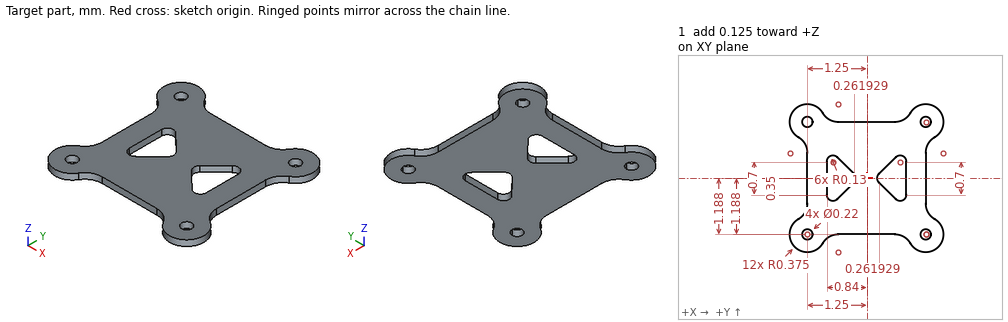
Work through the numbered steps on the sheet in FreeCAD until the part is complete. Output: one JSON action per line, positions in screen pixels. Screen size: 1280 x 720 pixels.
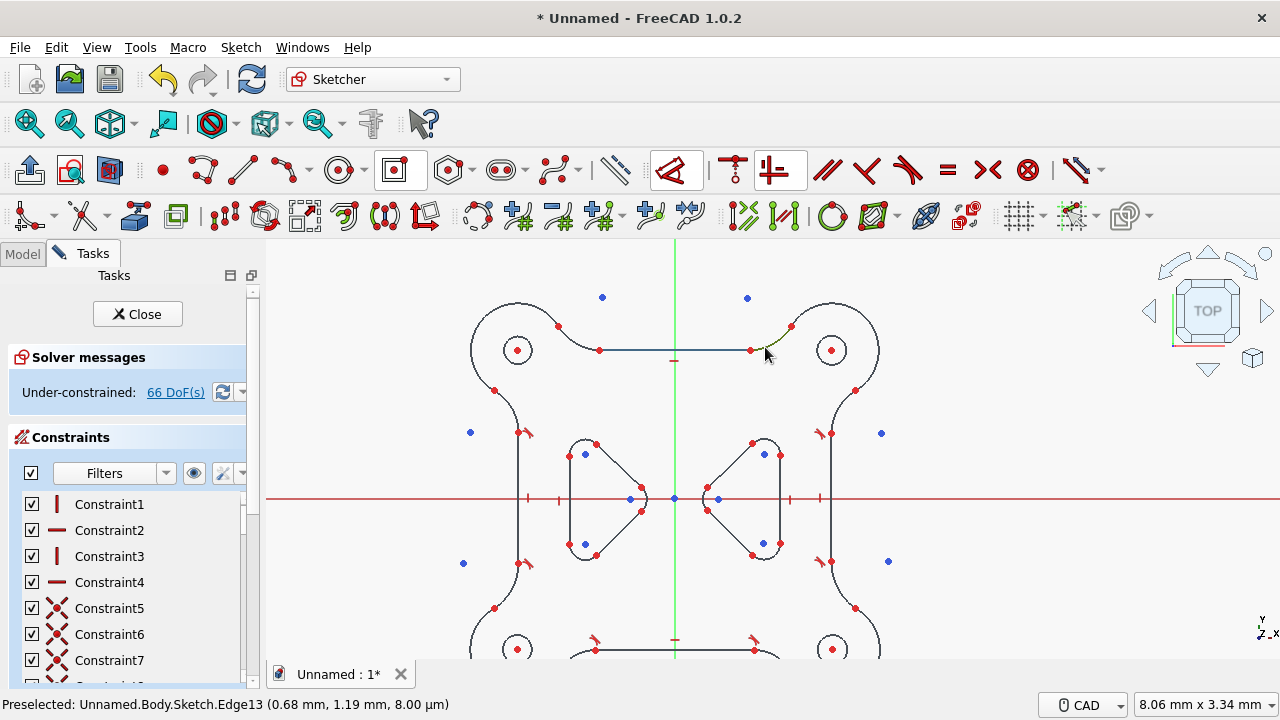
{"action": "left_click", "coordinate": [908, 170]}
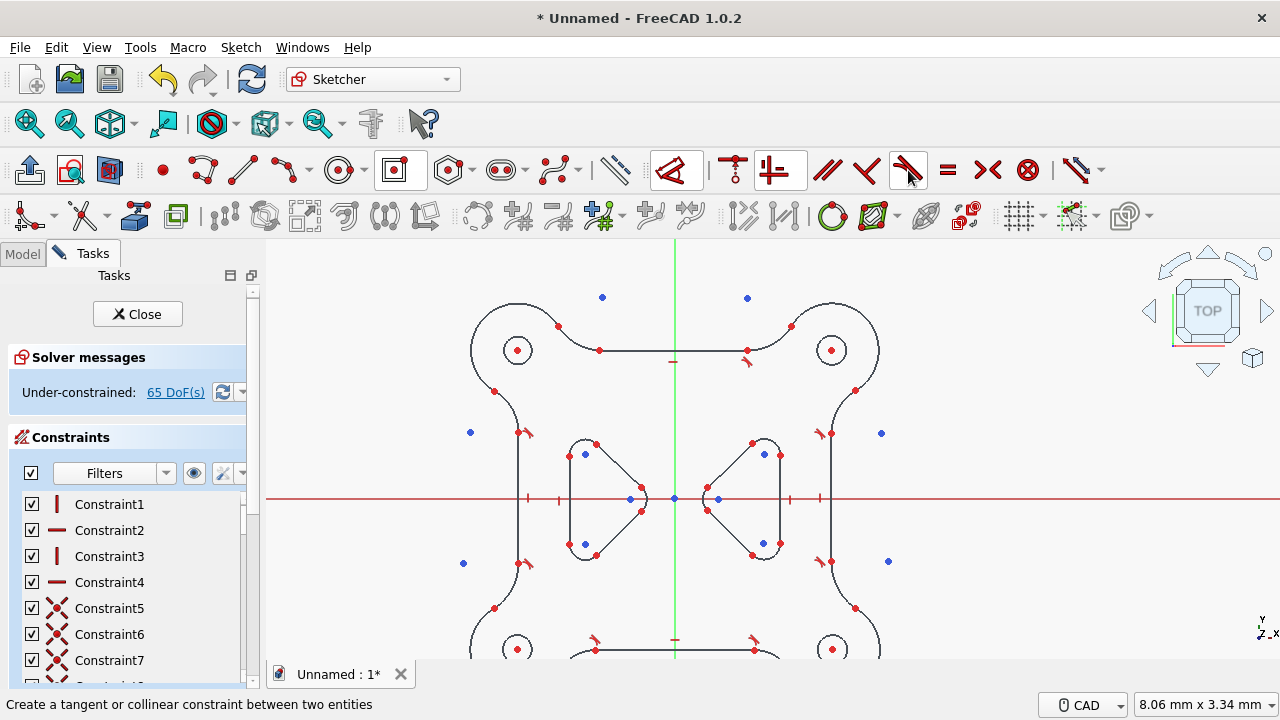
{"action": "left_click", "coordinate": [703, 351]}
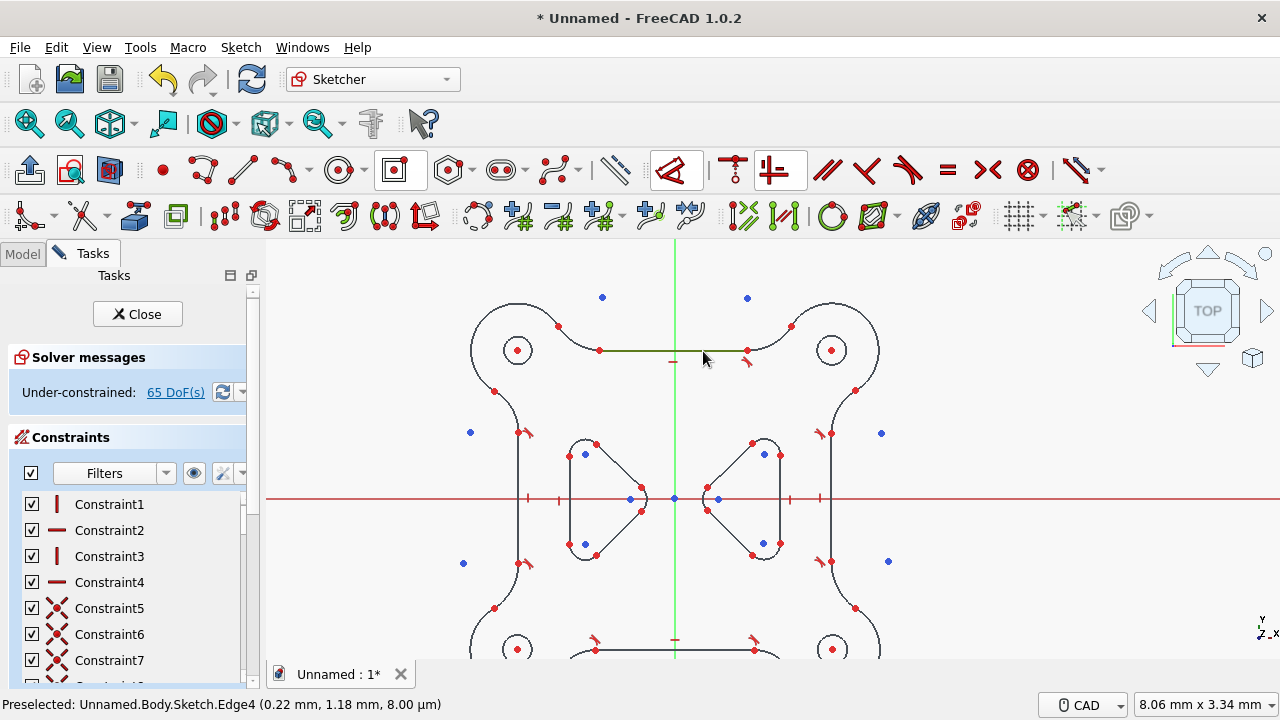
{"action": "left_click", "coordinate": [568, 338]}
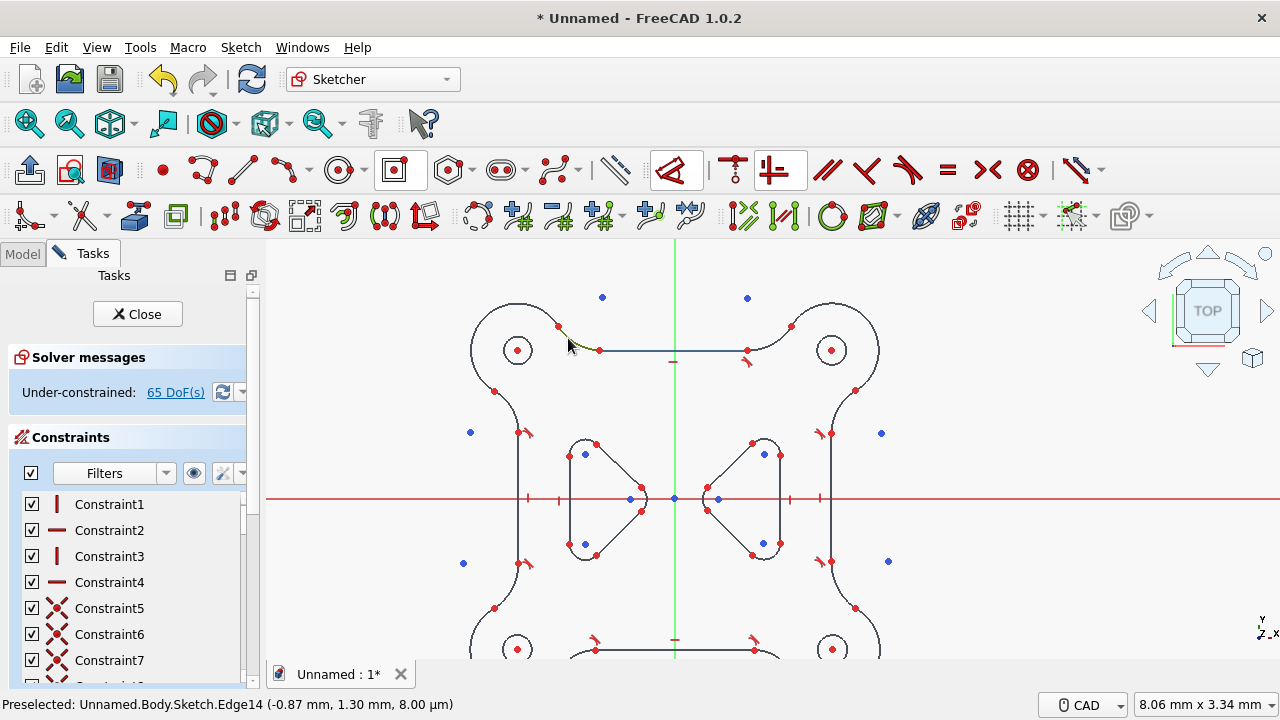
{"action": "left_click", "coordinate": [908, 170]}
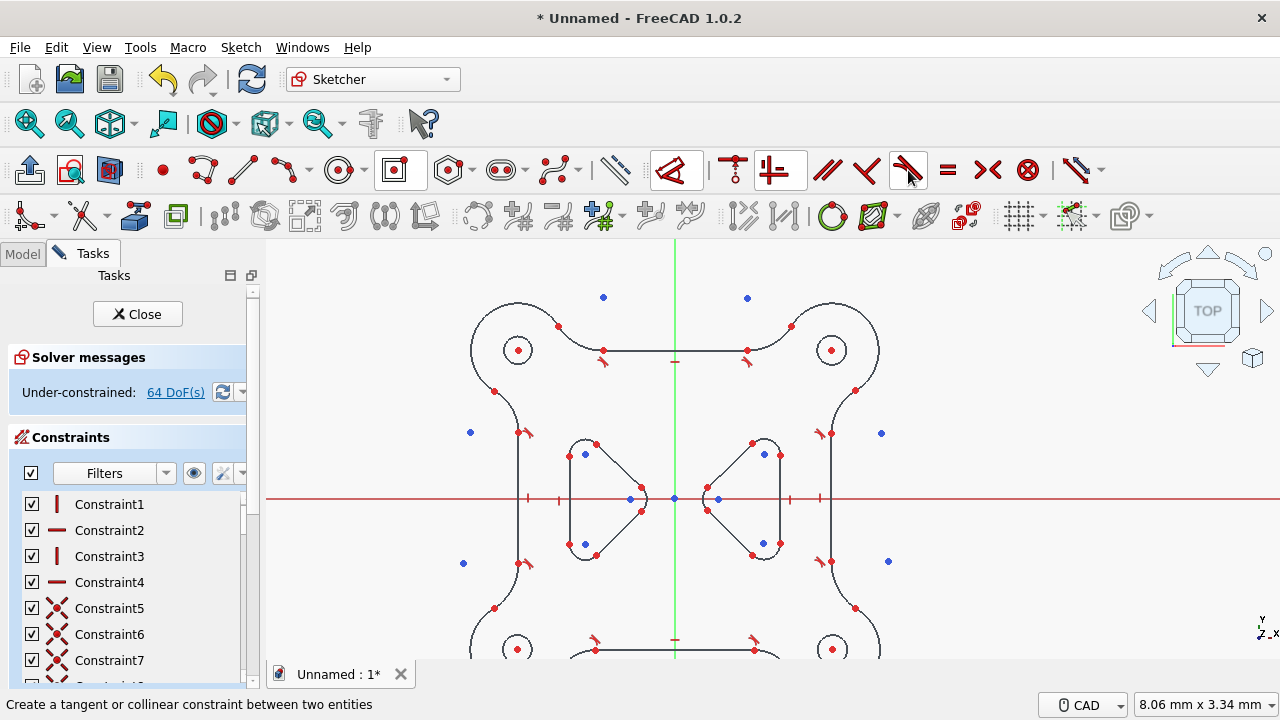
{"action": "left_click", "coordinate": [506, 598]}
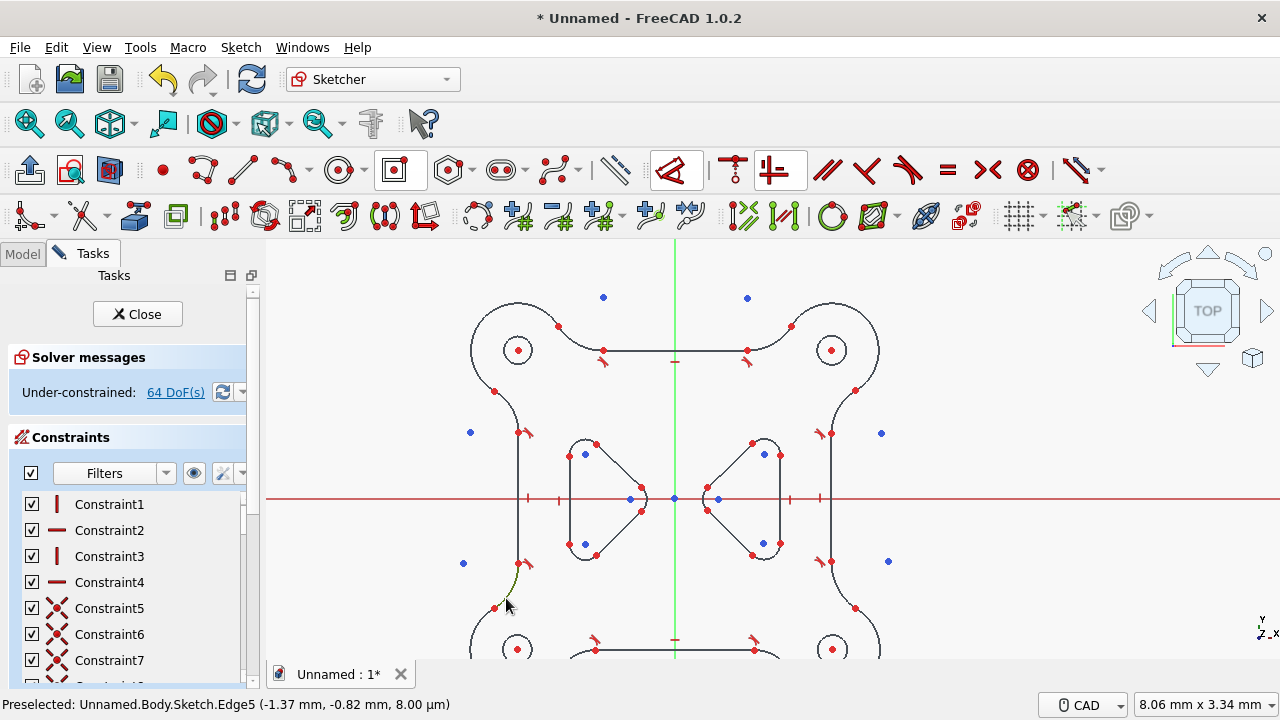
{"action": "scroll", "coordinate": [765, 348], "scroll_direction": "down", "scroll_amount": 2}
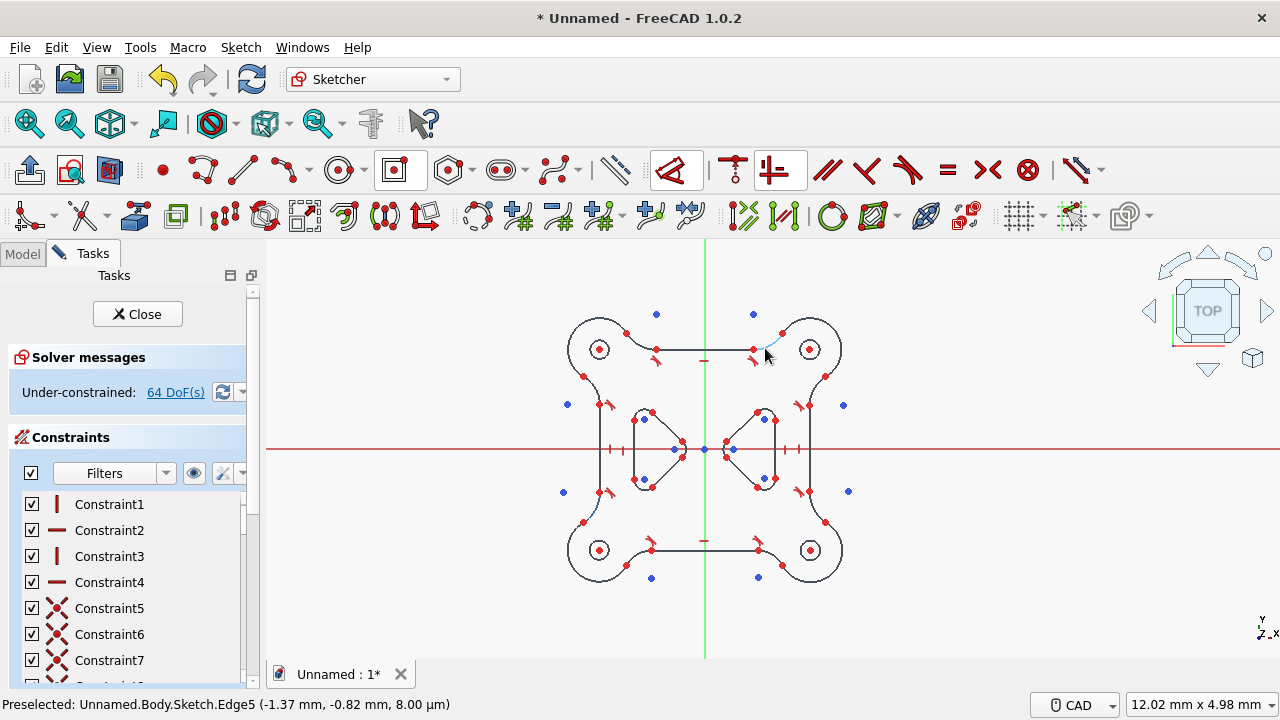
{"action": "left_click", "coordinate": [568, 552]}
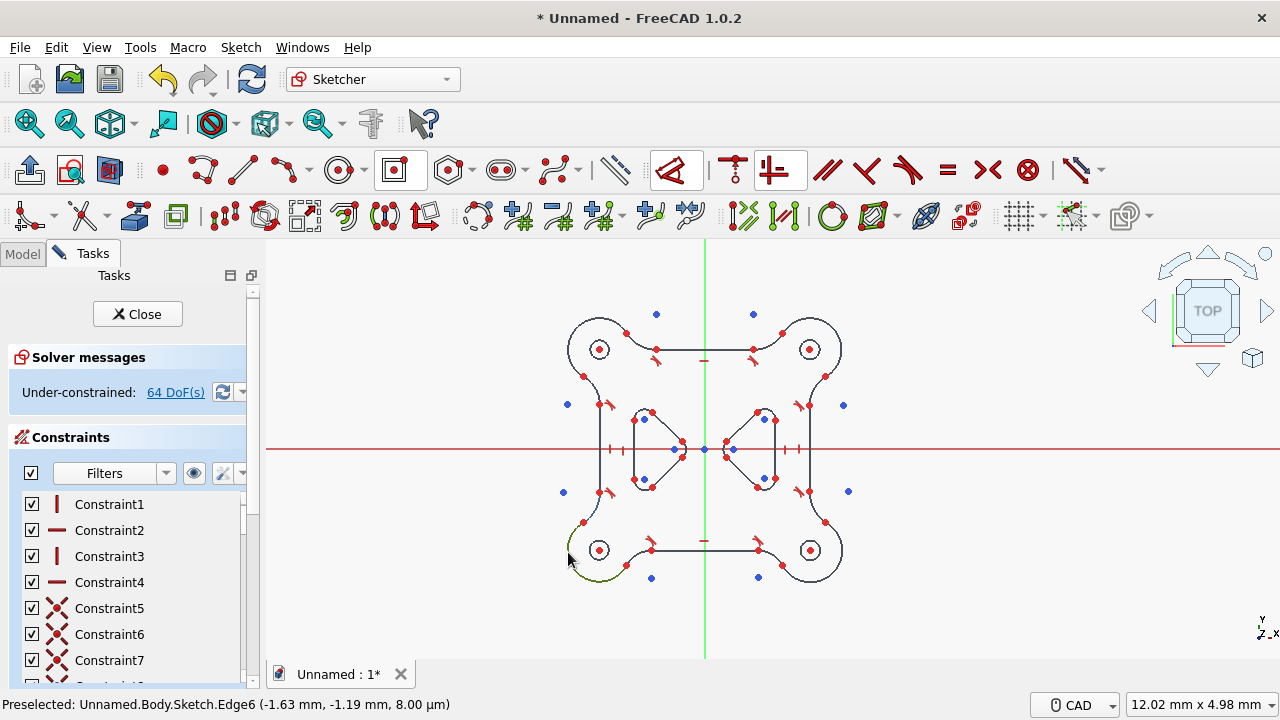
{"action": "left_click", "coordinate": [908, 170]}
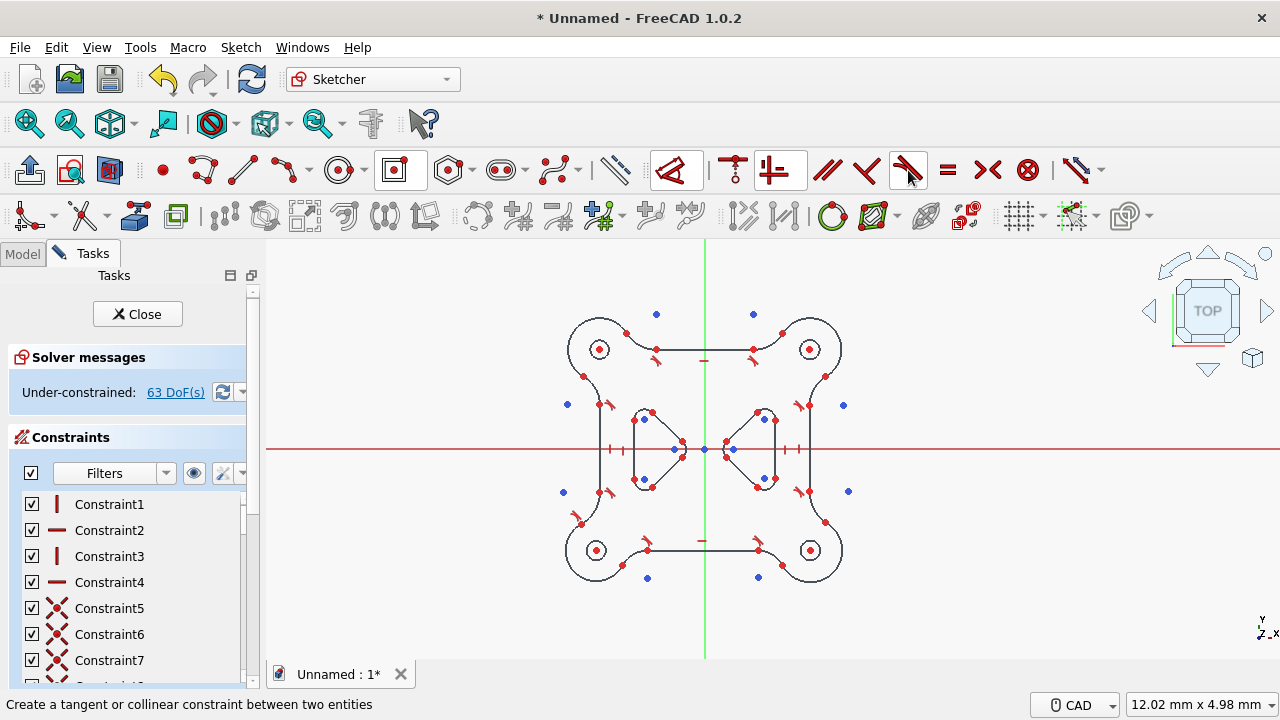
{"action": "left_click", "coordinate": [566, 552]}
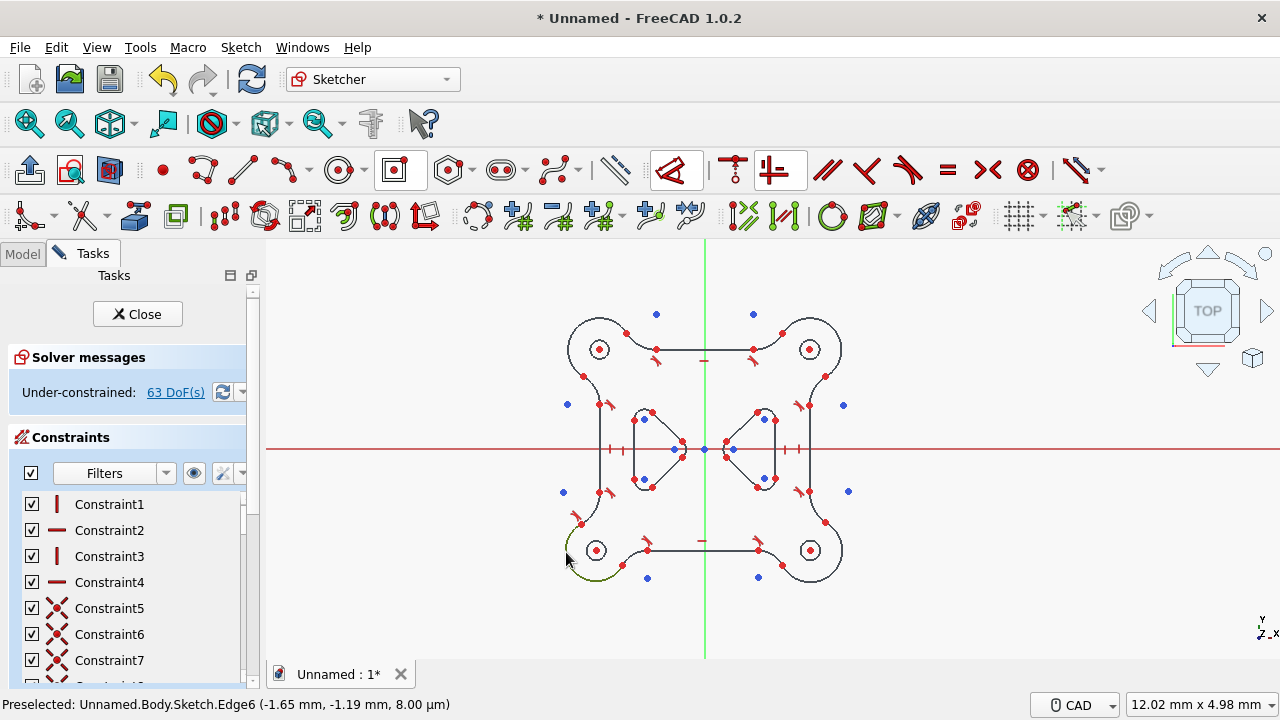
{"action": "scroll", "coordinate": [639, 552], "scroll_direction": "up", "scroll_amount": 3}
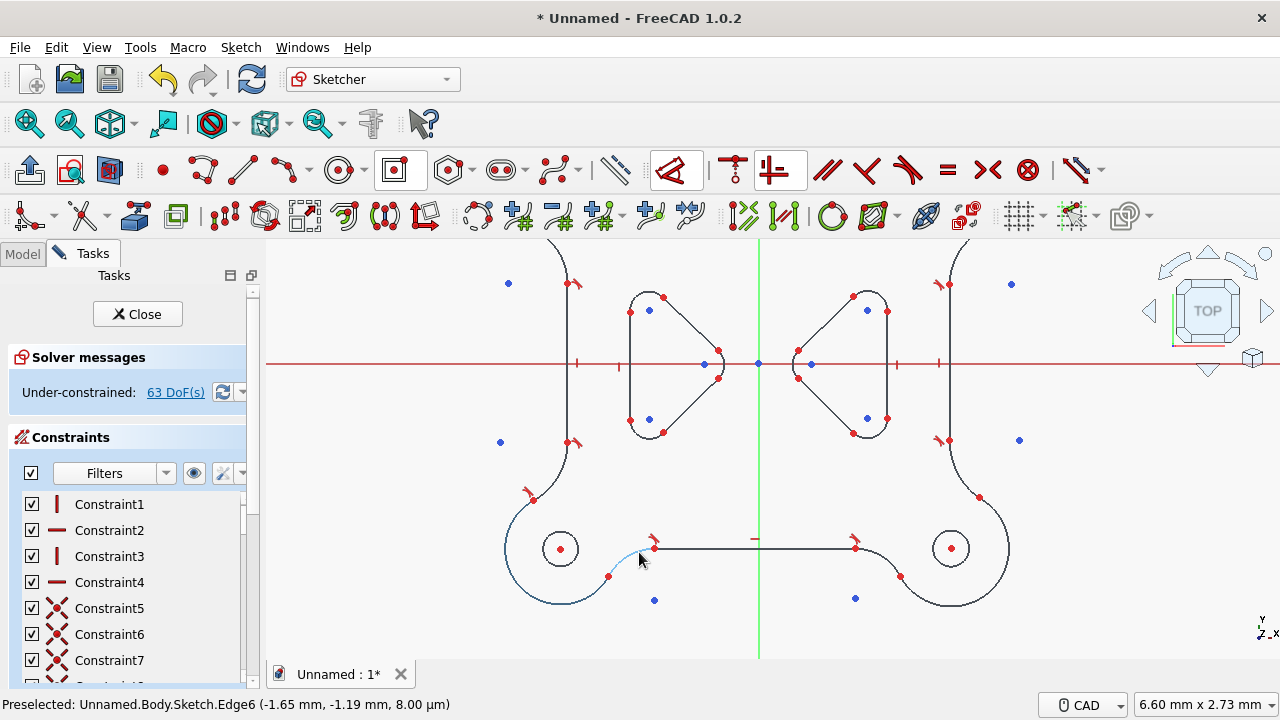
{"action": "left_click", "coordinate": [638, 552]}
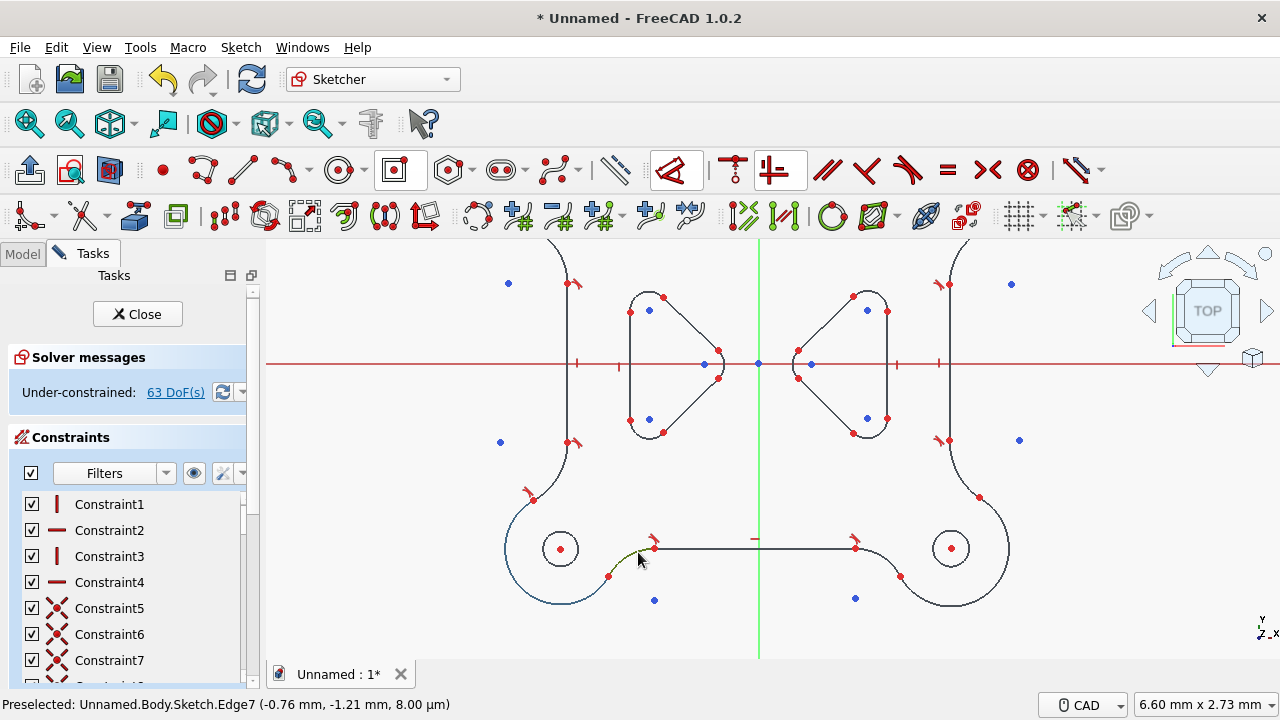
{"action": "left_click", "coordinate": [908, 170]}